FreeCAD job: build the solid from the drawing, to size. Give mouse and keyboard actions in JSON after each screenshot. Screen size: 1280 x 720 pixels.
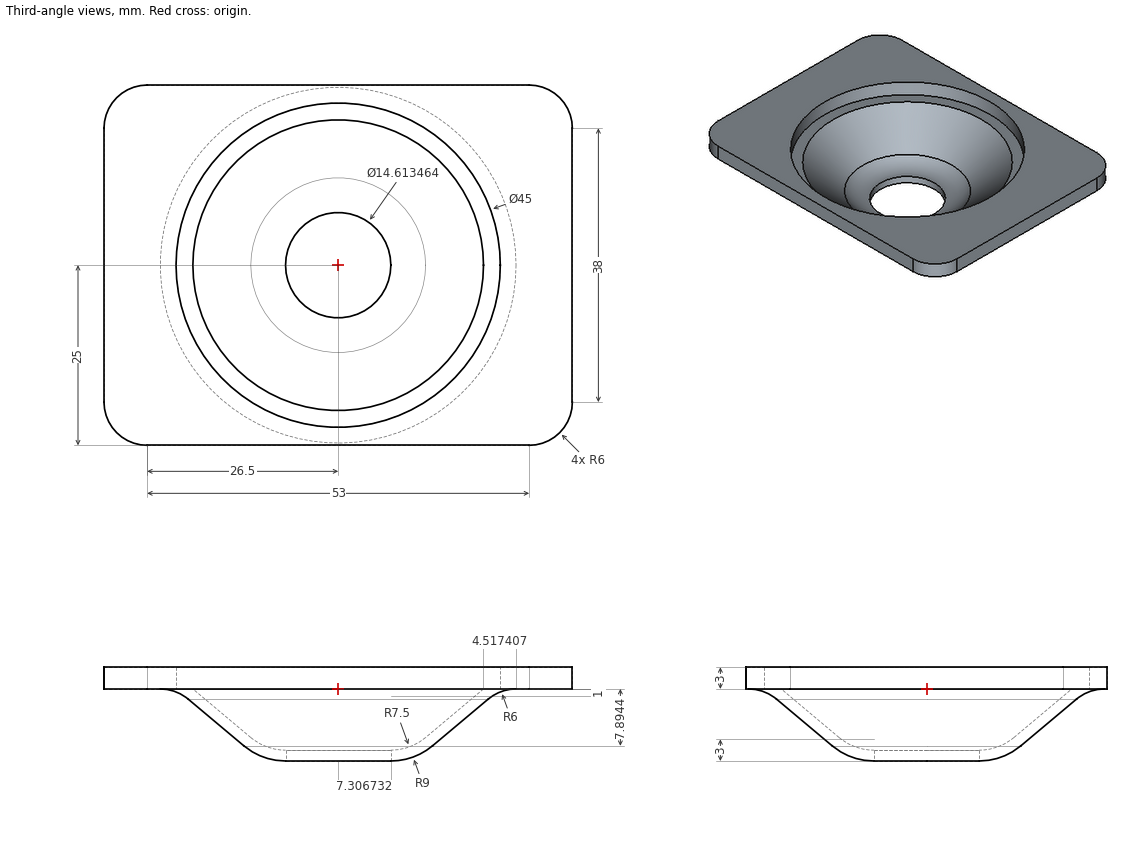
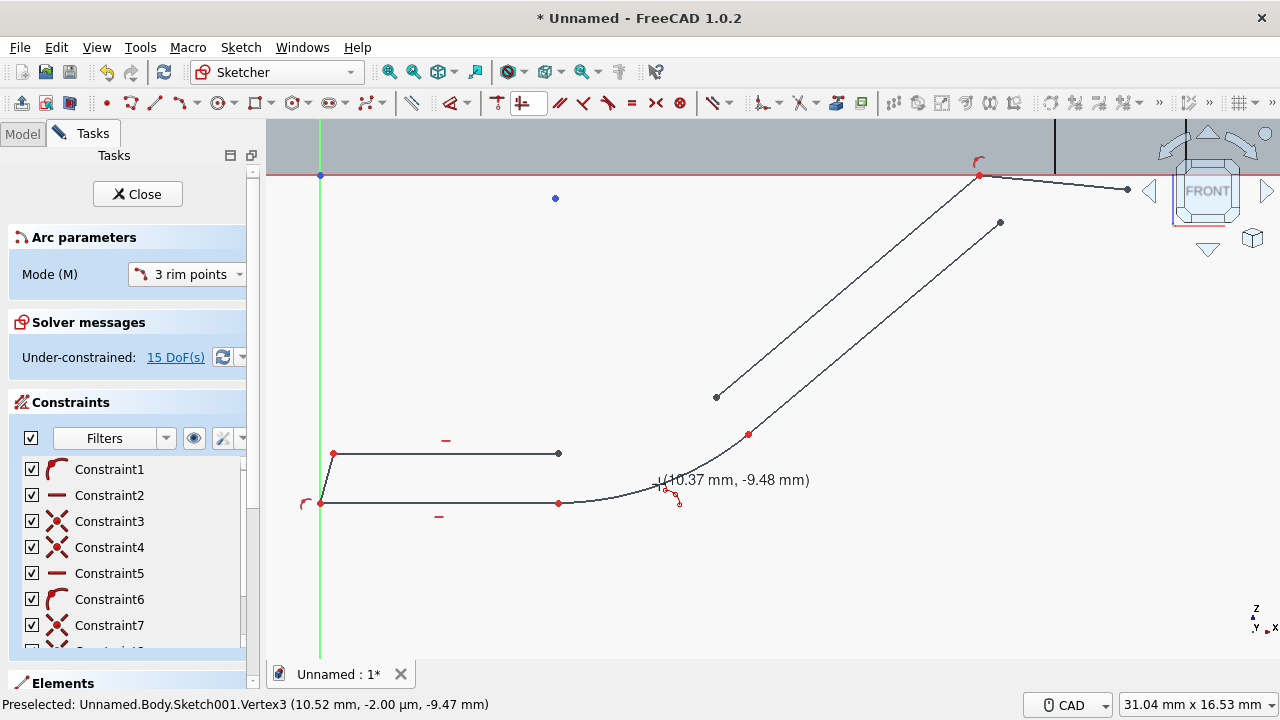
{"action": "left_click", "coordinate": [559, 454]}
{"action": "left_click", "coordinate": [717, 397]}
{"action": "left_click", "coordinate": [643, 438]}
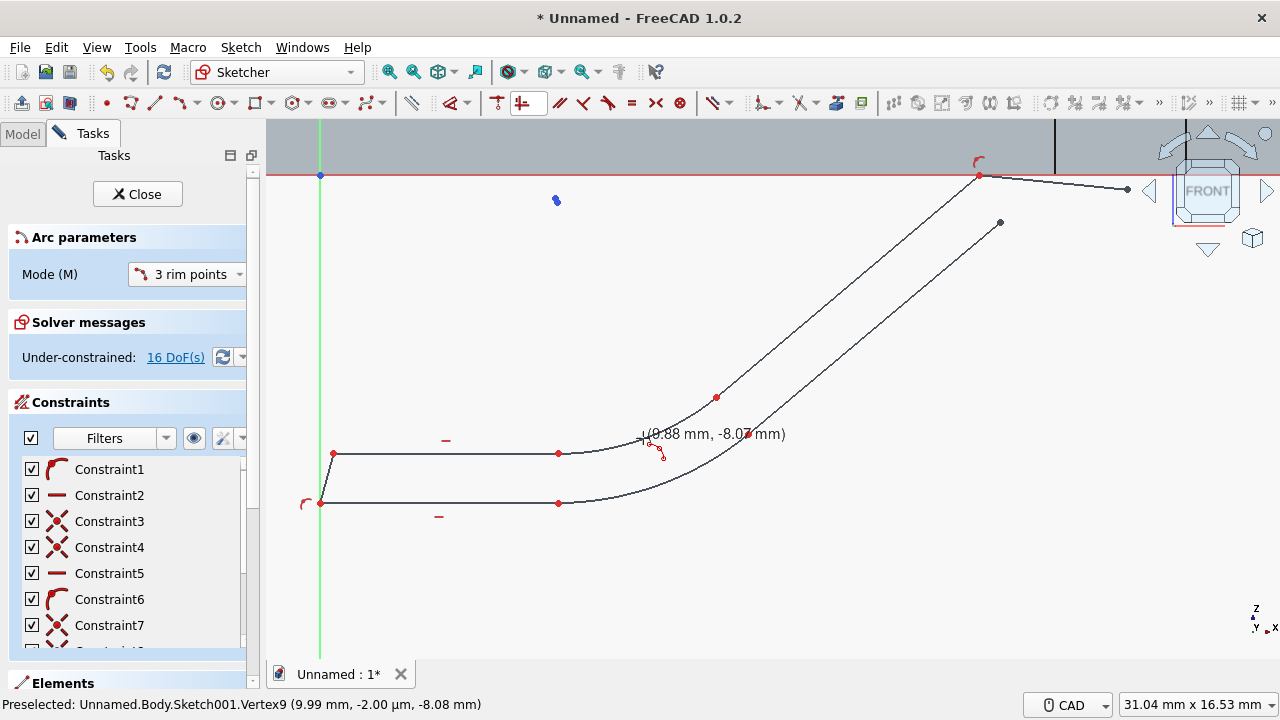
{"action": "scroll", "coordinate": [666, 491], "scroll_direction": "down", "scroll_amount": 2}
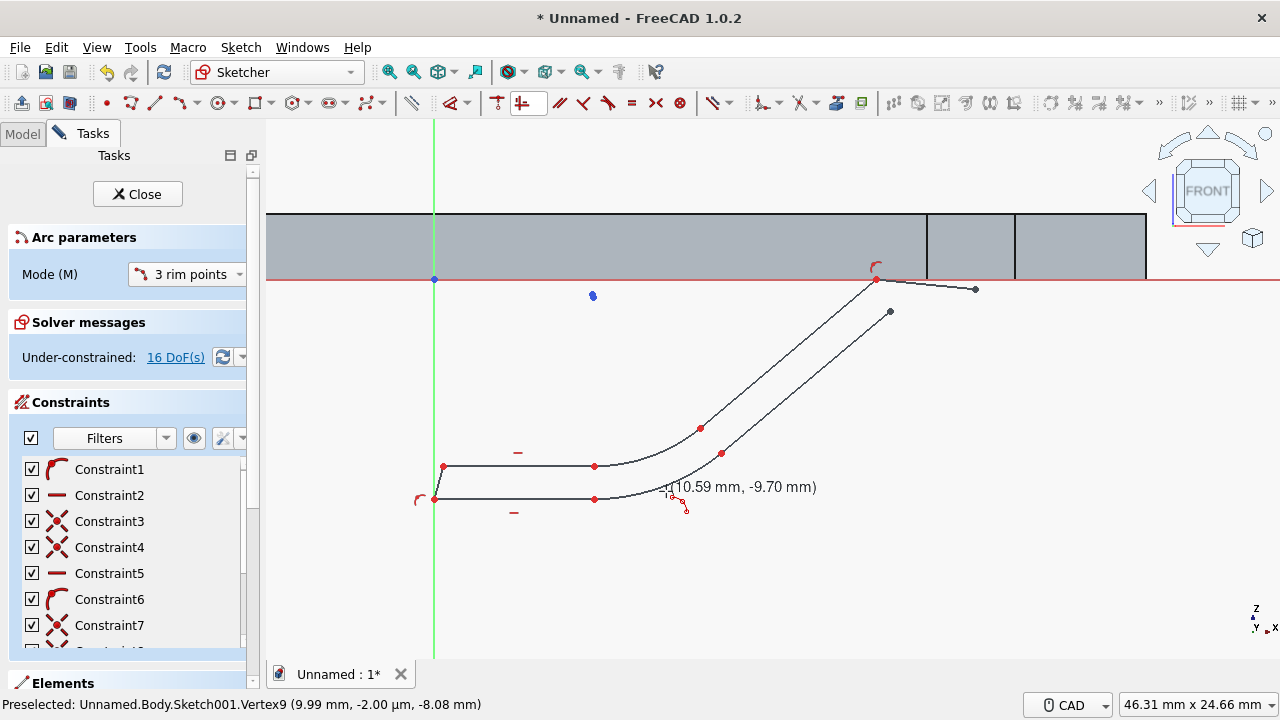
{"action": "left_click", "coordinate": [975, 289]}
{"action": "left_click", "coordinate": [890, 311]}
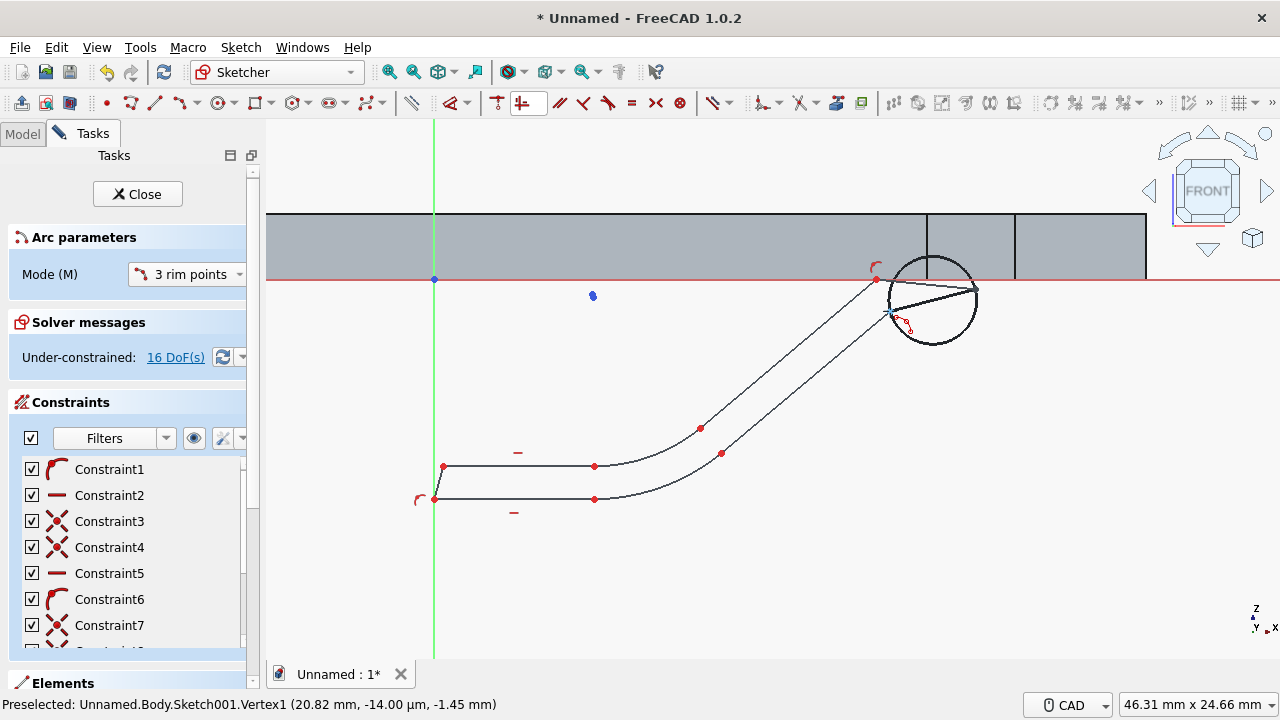
{"action": "scroll", "coordinate": [930, 288], "scroll_direction": "up", "scroll_amount": 4}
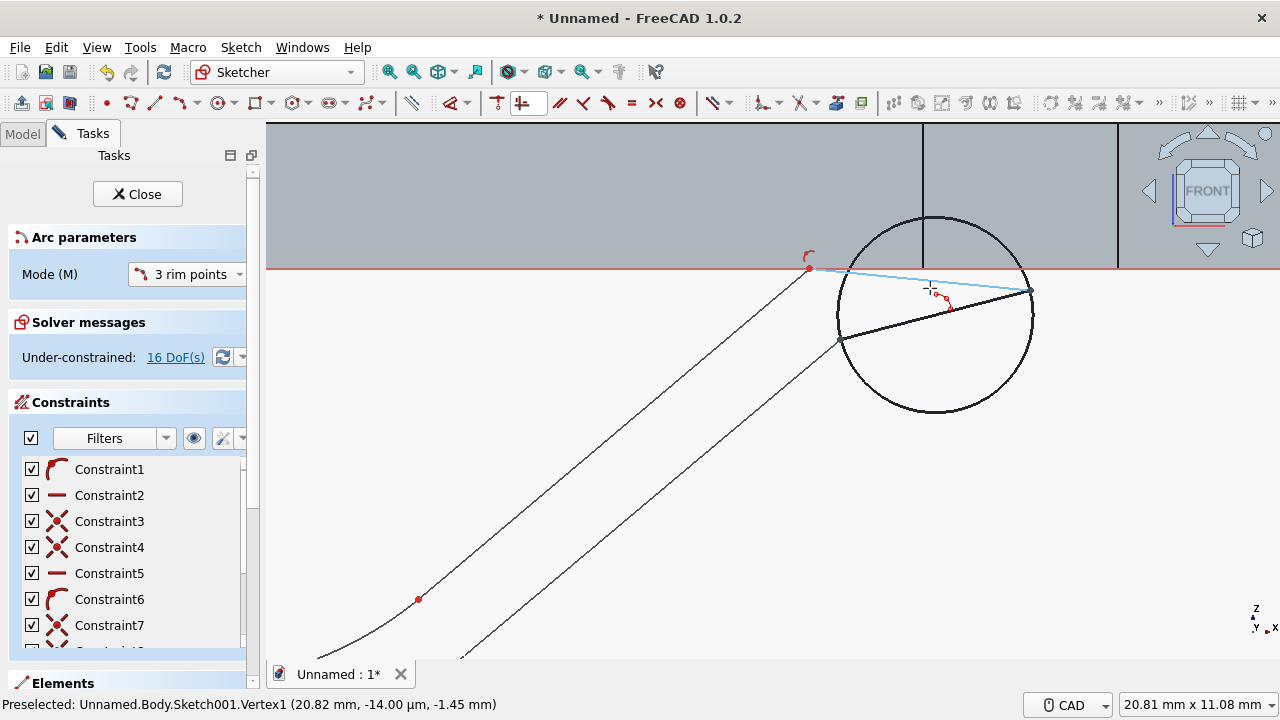
{"action": "left_click", "coordinate": [929, 287]}
{"action": "key", "text": "Escape"}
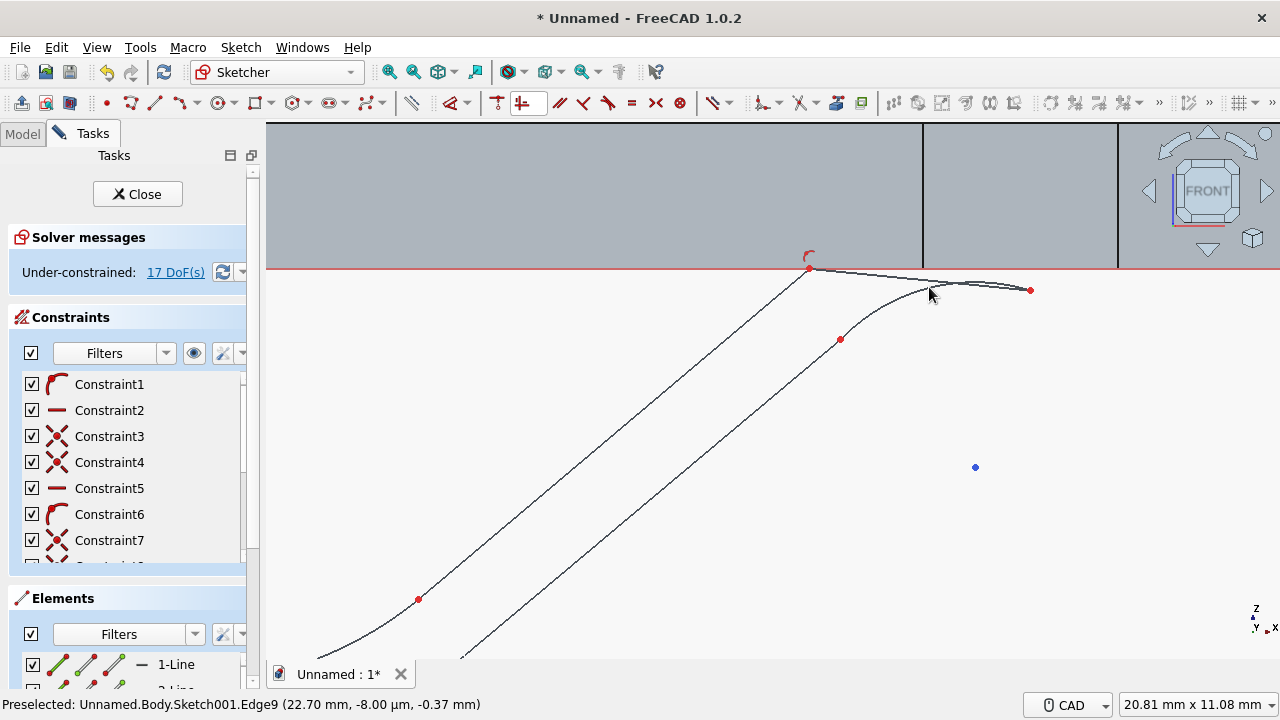
{"action": "left_click", "coordinate": [728, 434]}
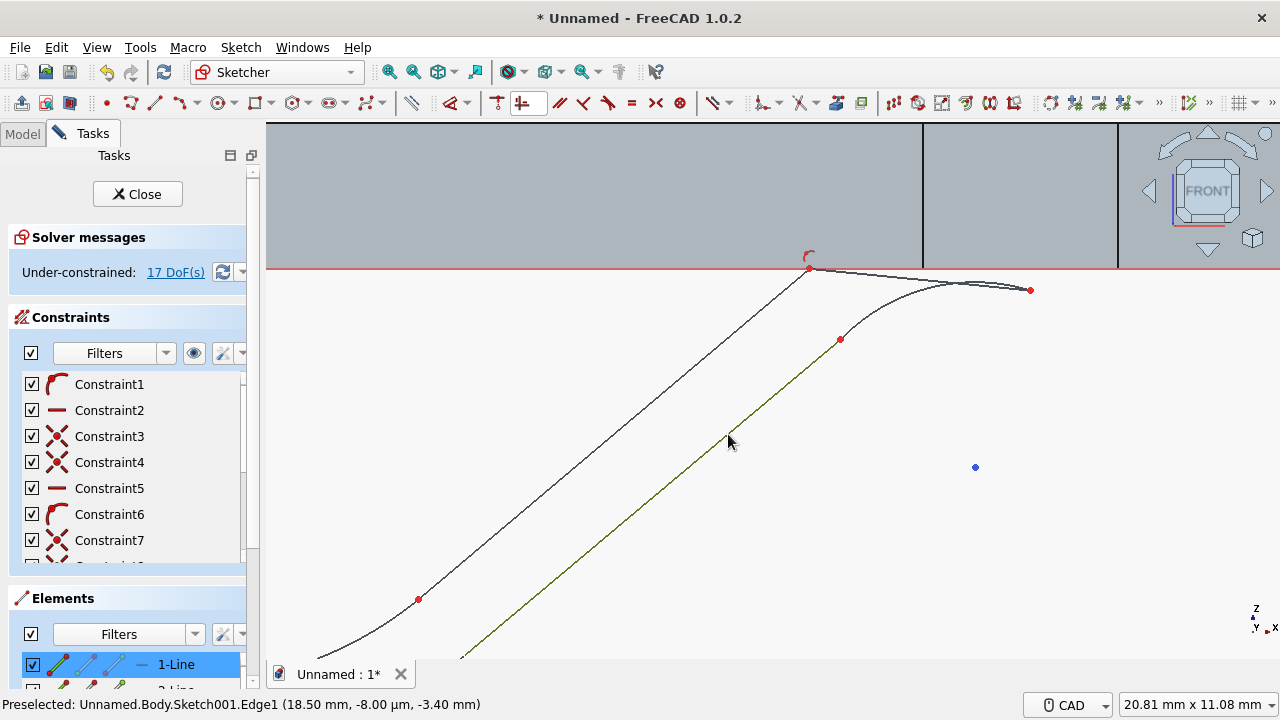
{"action": "scroll", "coordinate": [931, 288], "scroll_direction": "down", "scroll_amount": 4}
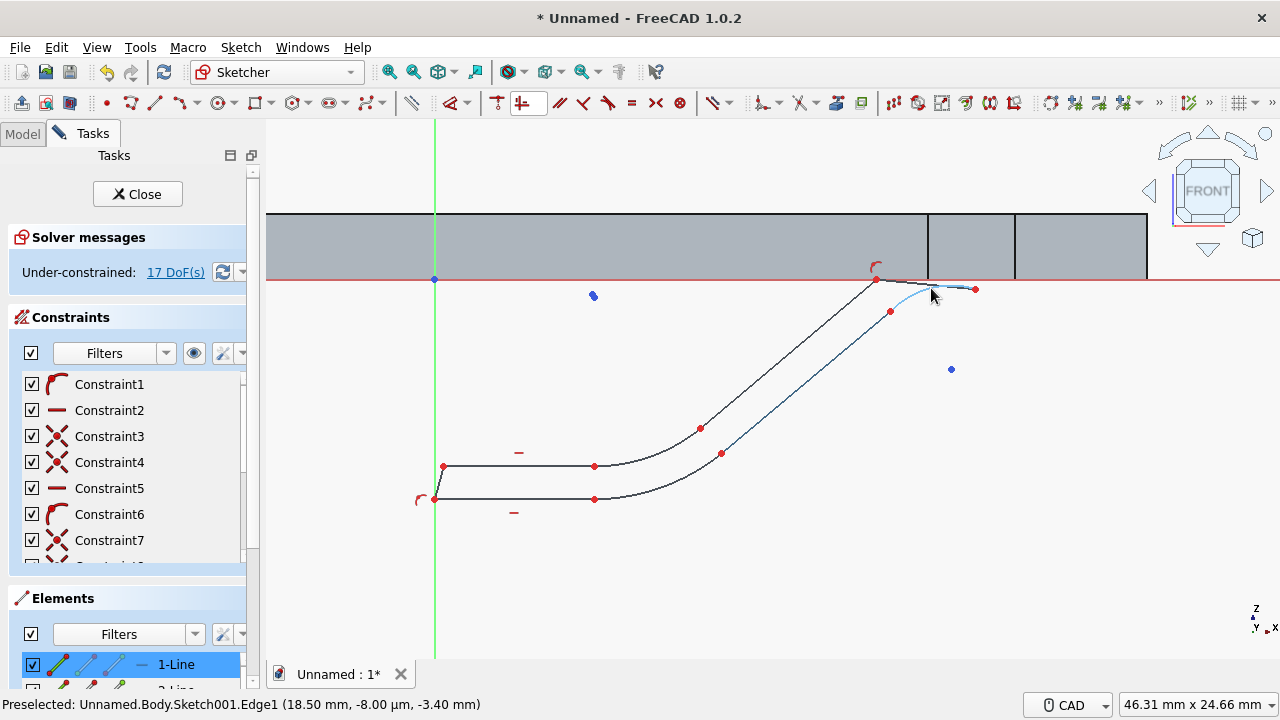
{"action": "left_click", "coordinate": [636, 495]}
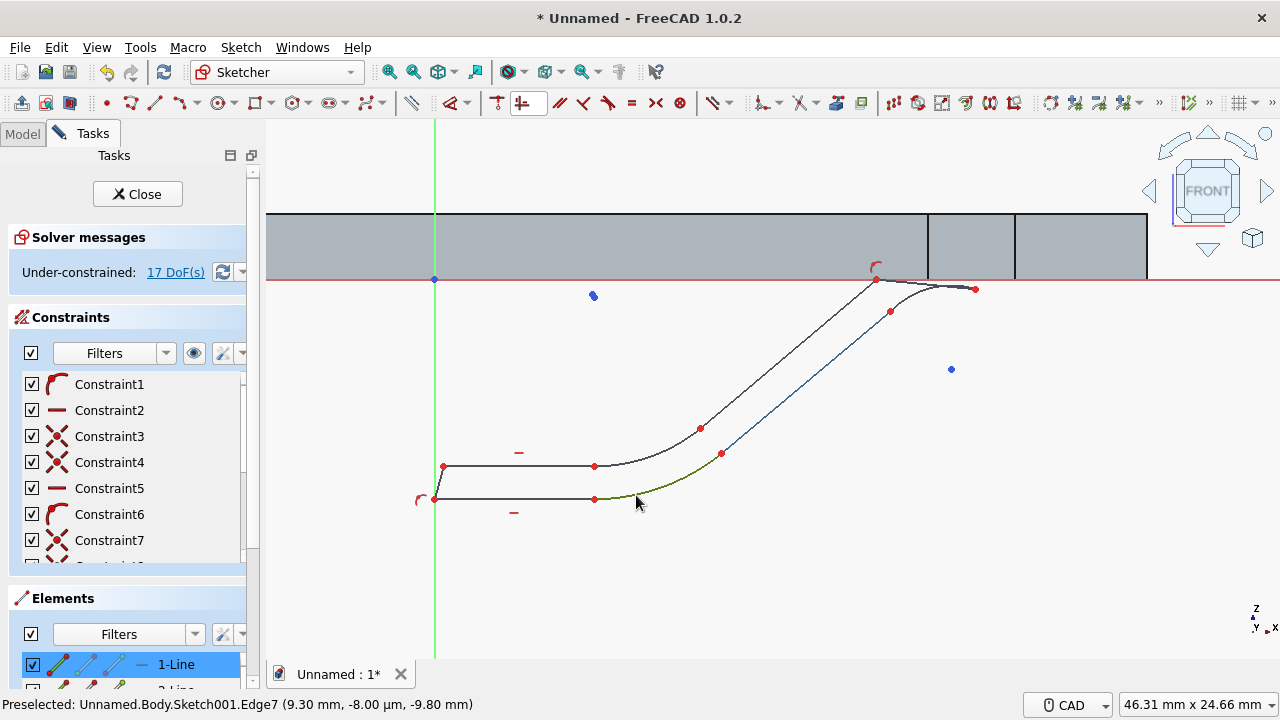
{"action": "left_click", "coordinate": [608, 104]}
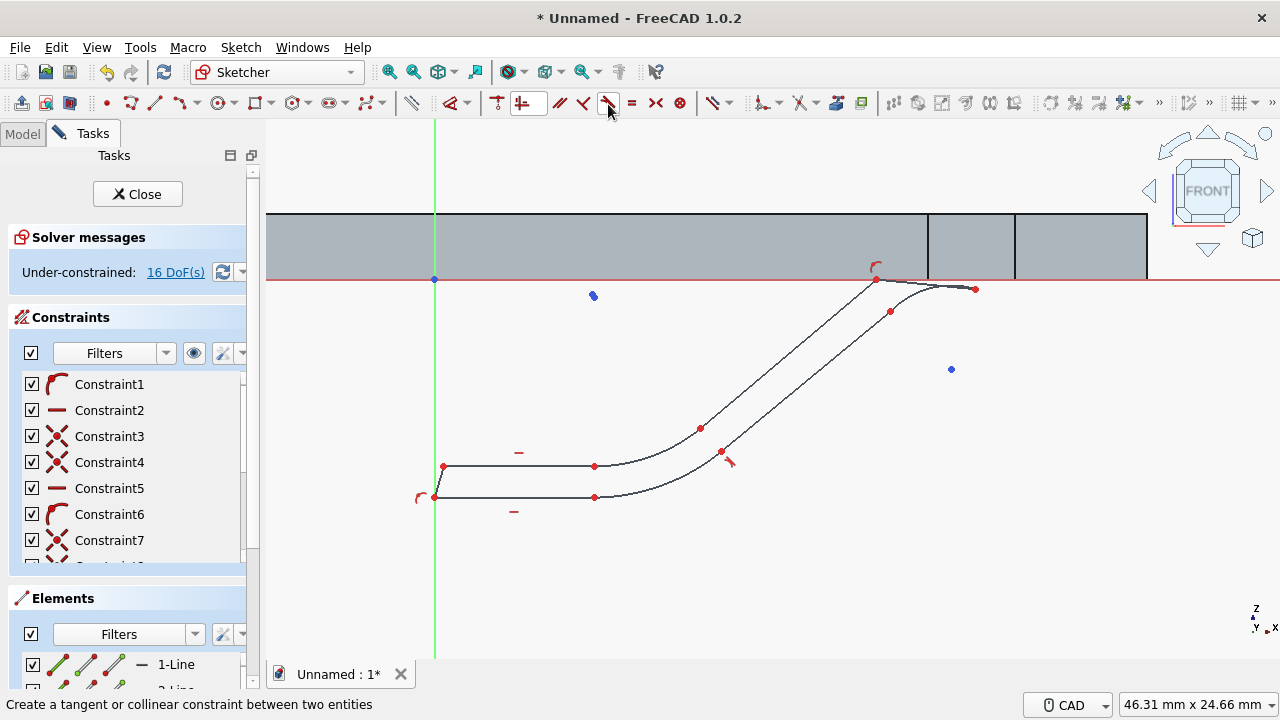
{"action": "left_click", "coordinate": [840, 353]}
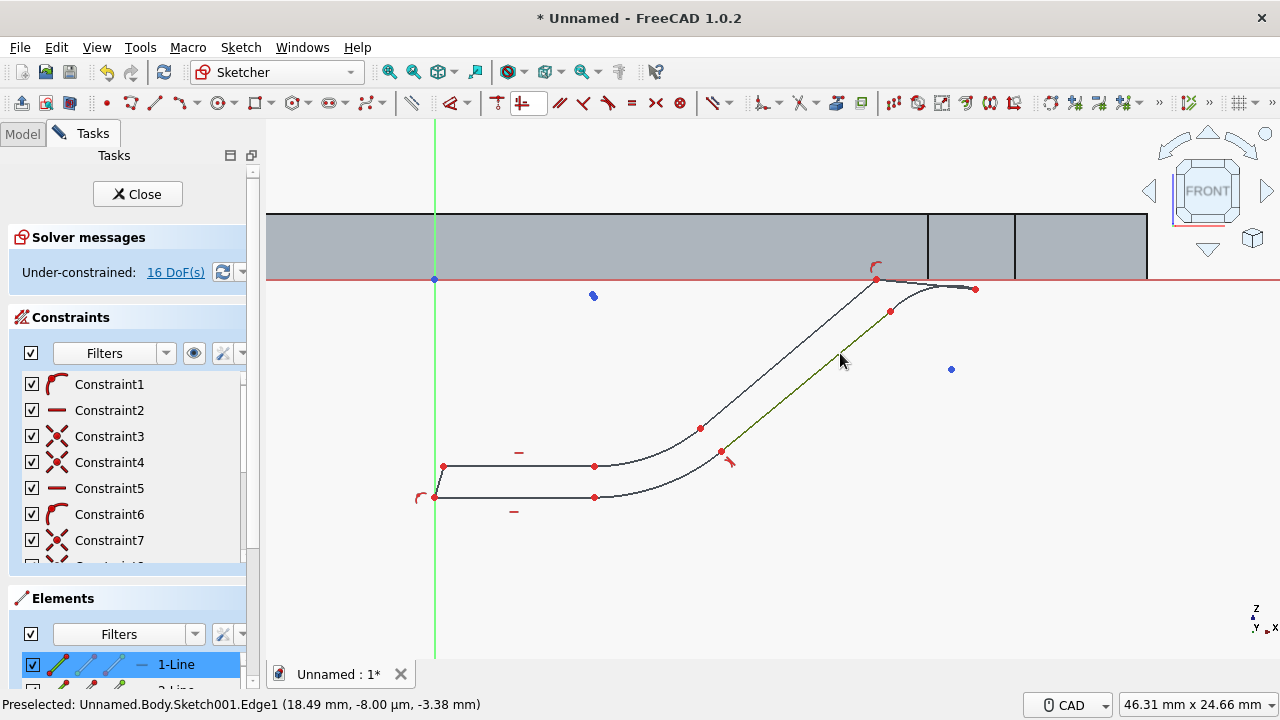
{"action": "left_click", "coordinate": [913, 295]}